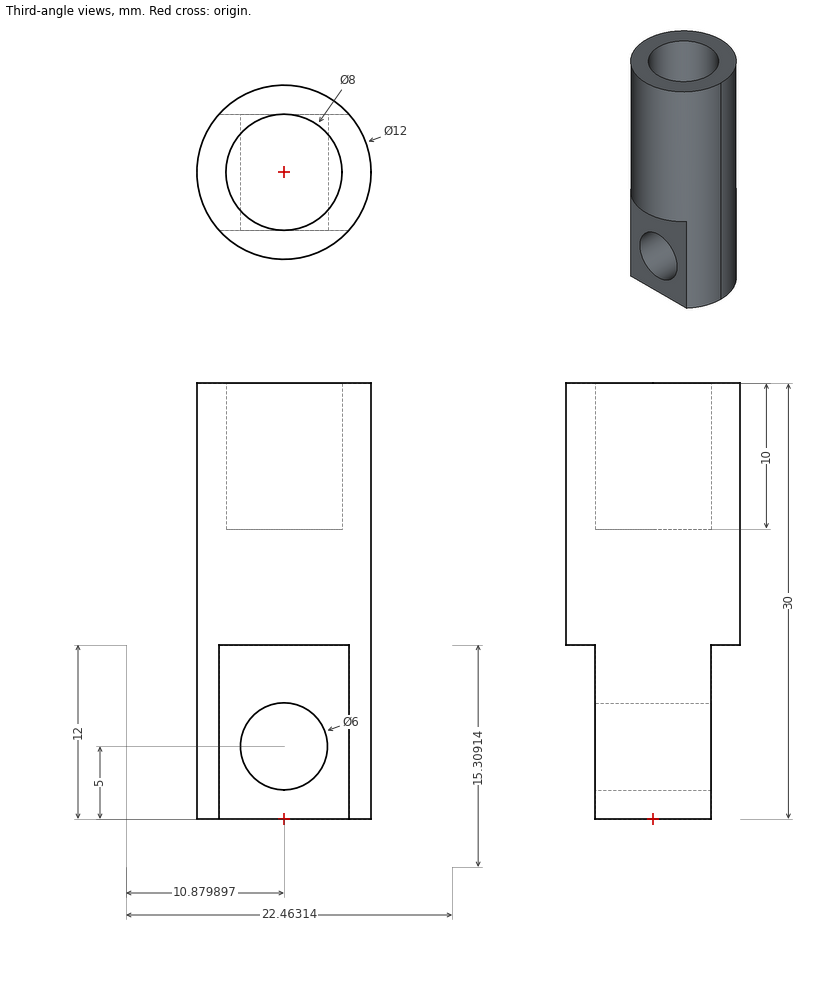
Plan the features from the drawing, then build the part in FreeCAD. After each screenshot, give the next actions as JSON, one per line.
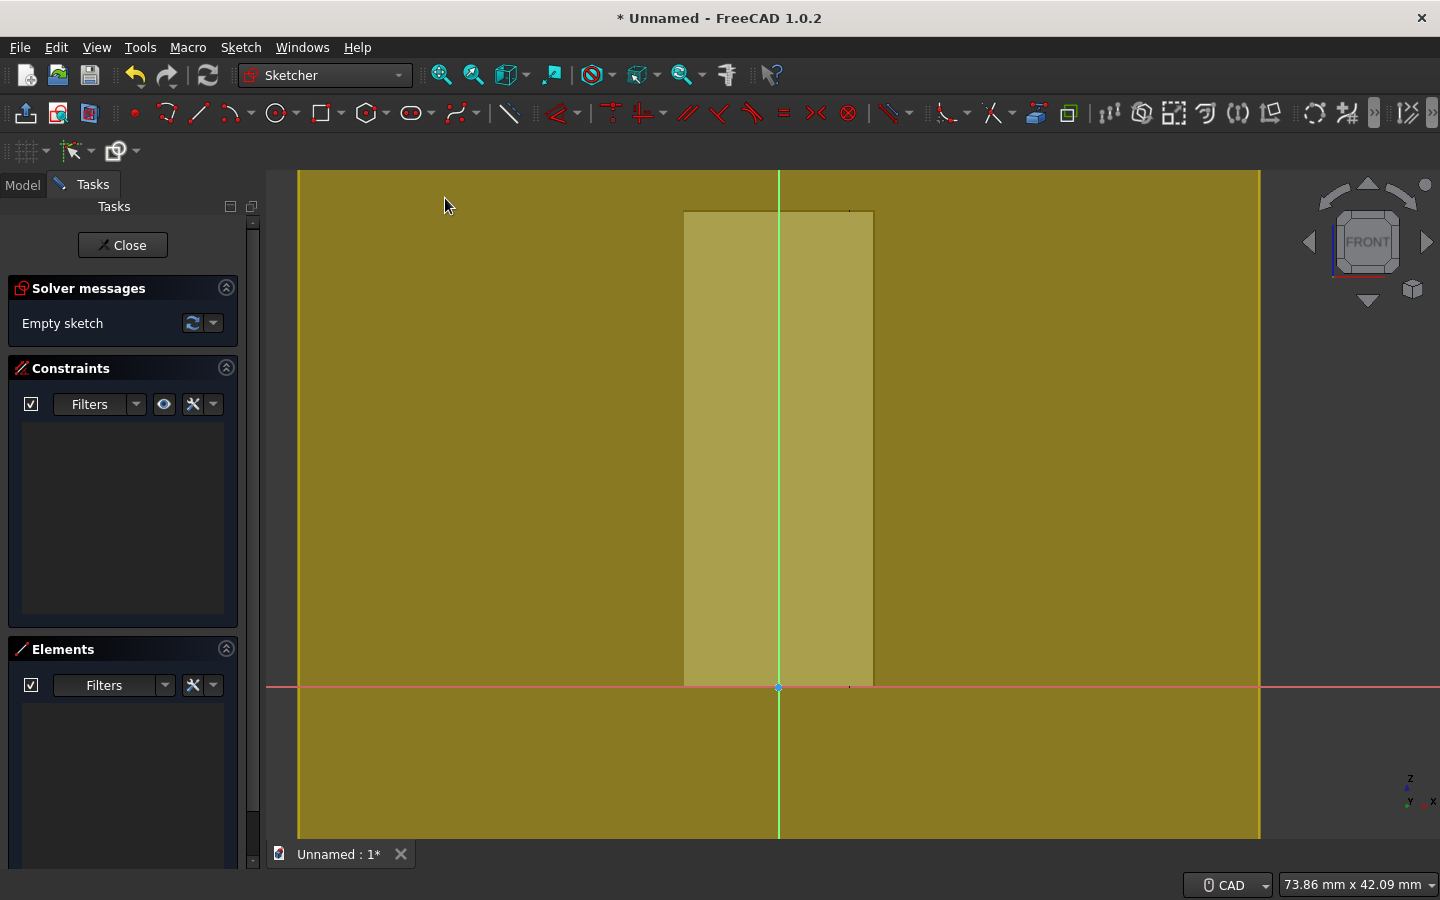
{"action": "scroll", "coordinate": [785, 757], "scroll_direction": "up", "scroll_amount": 3}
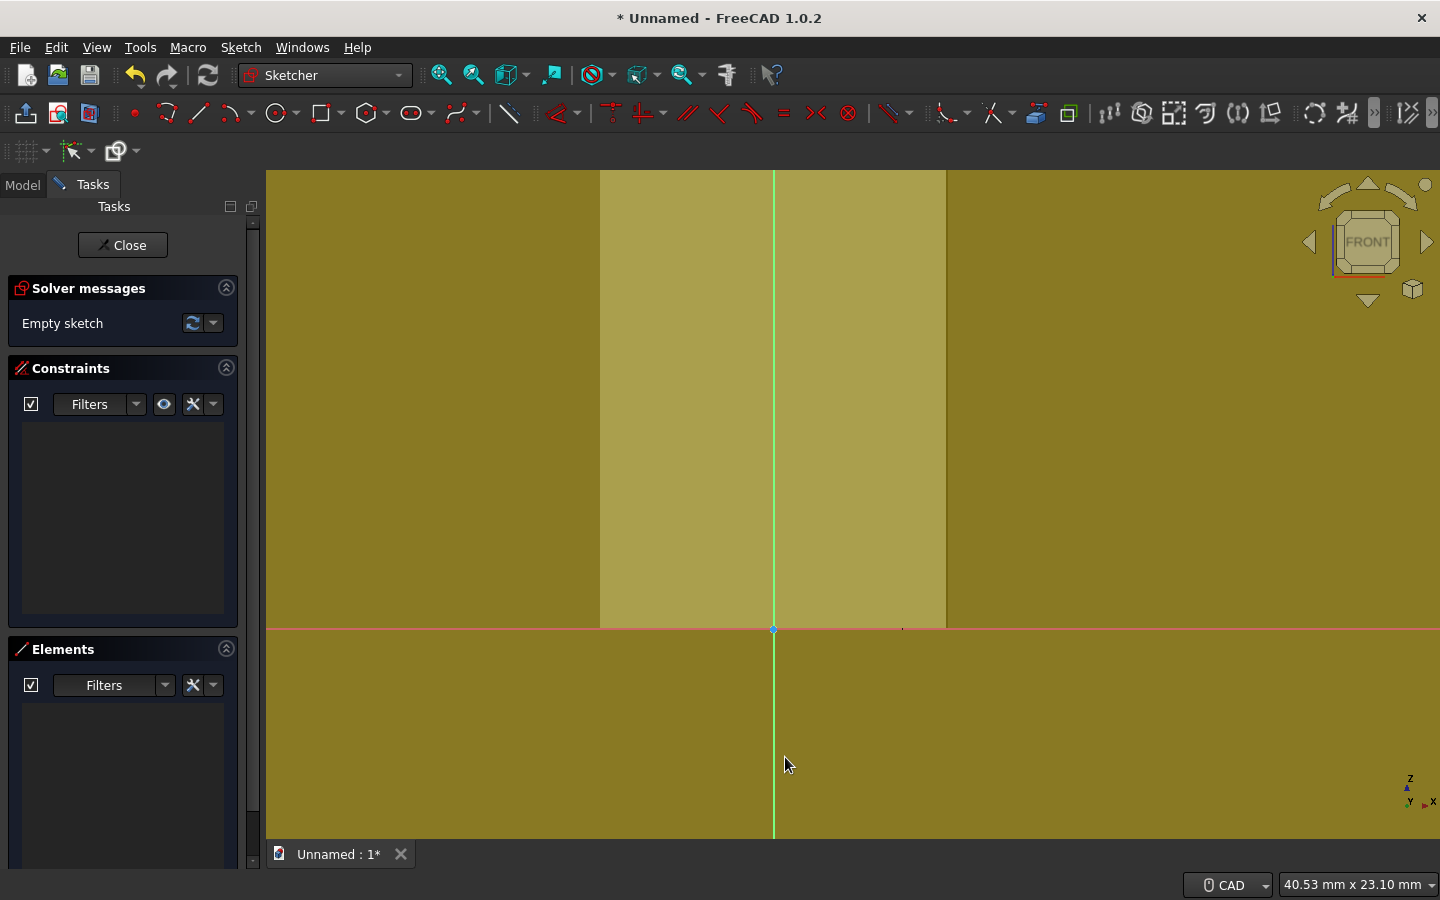
{"action": "left_click", "coordinate": [322, 114]}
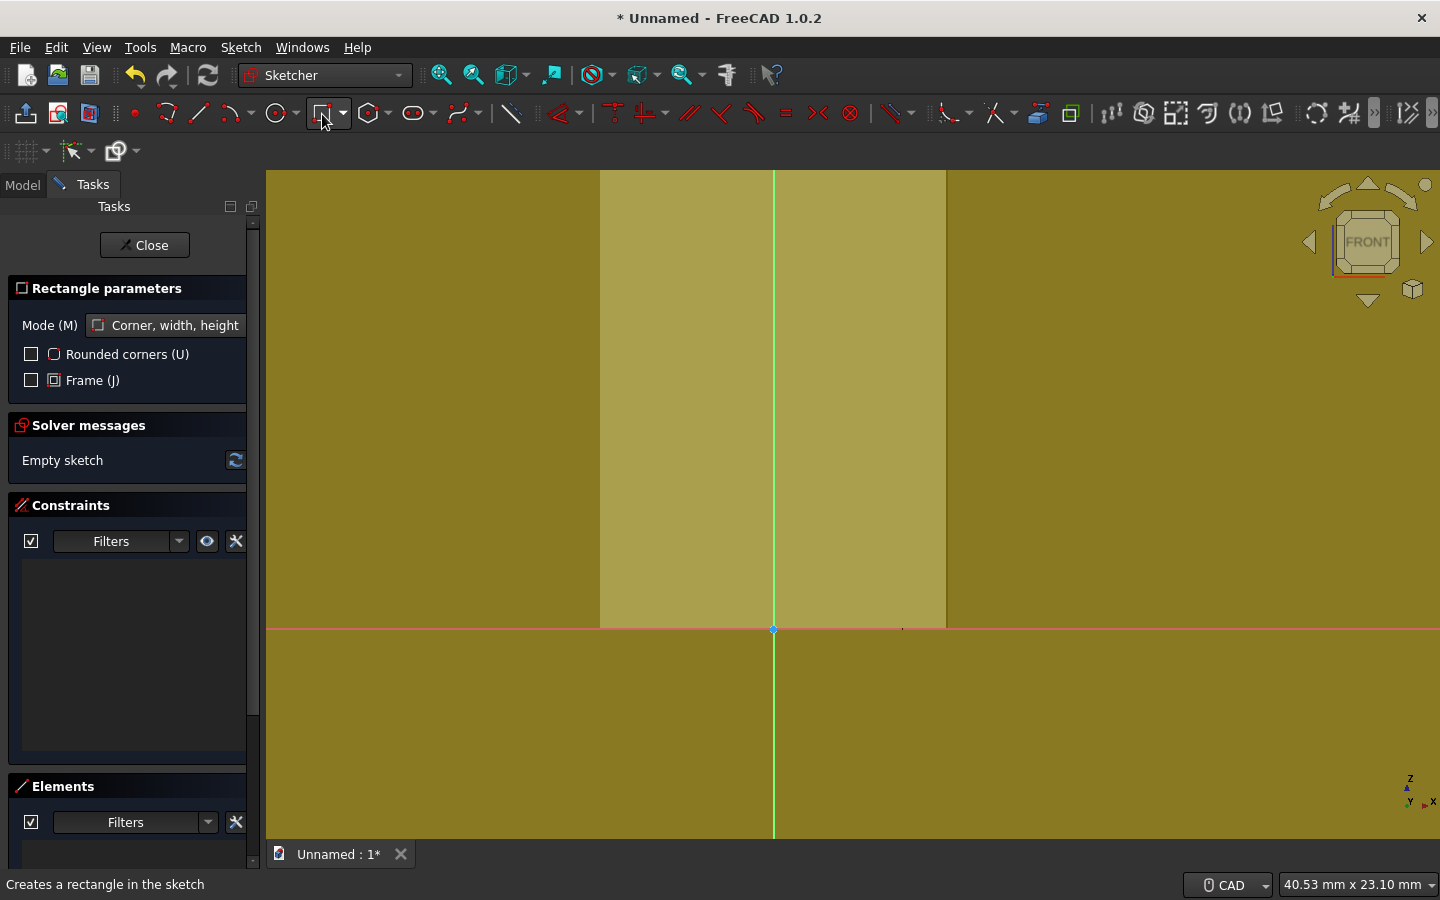
{"action": "left_click", "coordinate": [458, 282]}
{"action": "mouse_move", "coordinate": [1109, 725]}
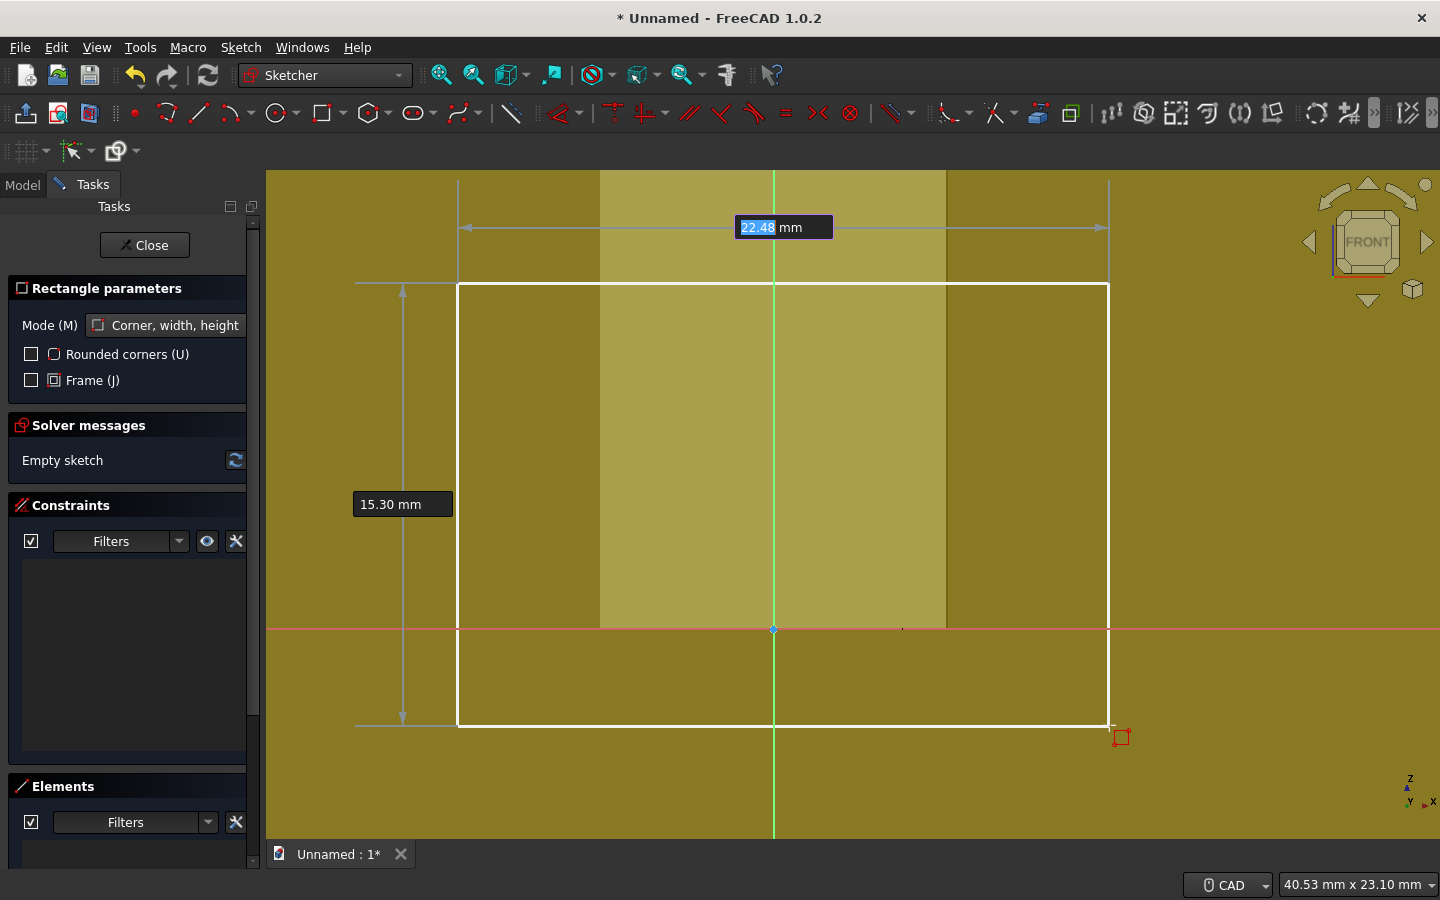
{"action": "type", "text": "22.46314"}
{"action": "key", "text": "Tab"}
{"action": "type", "text": "15.30914"}
{"action": "key", "text": "Return"}
{"action": "key", "text": "Escape"}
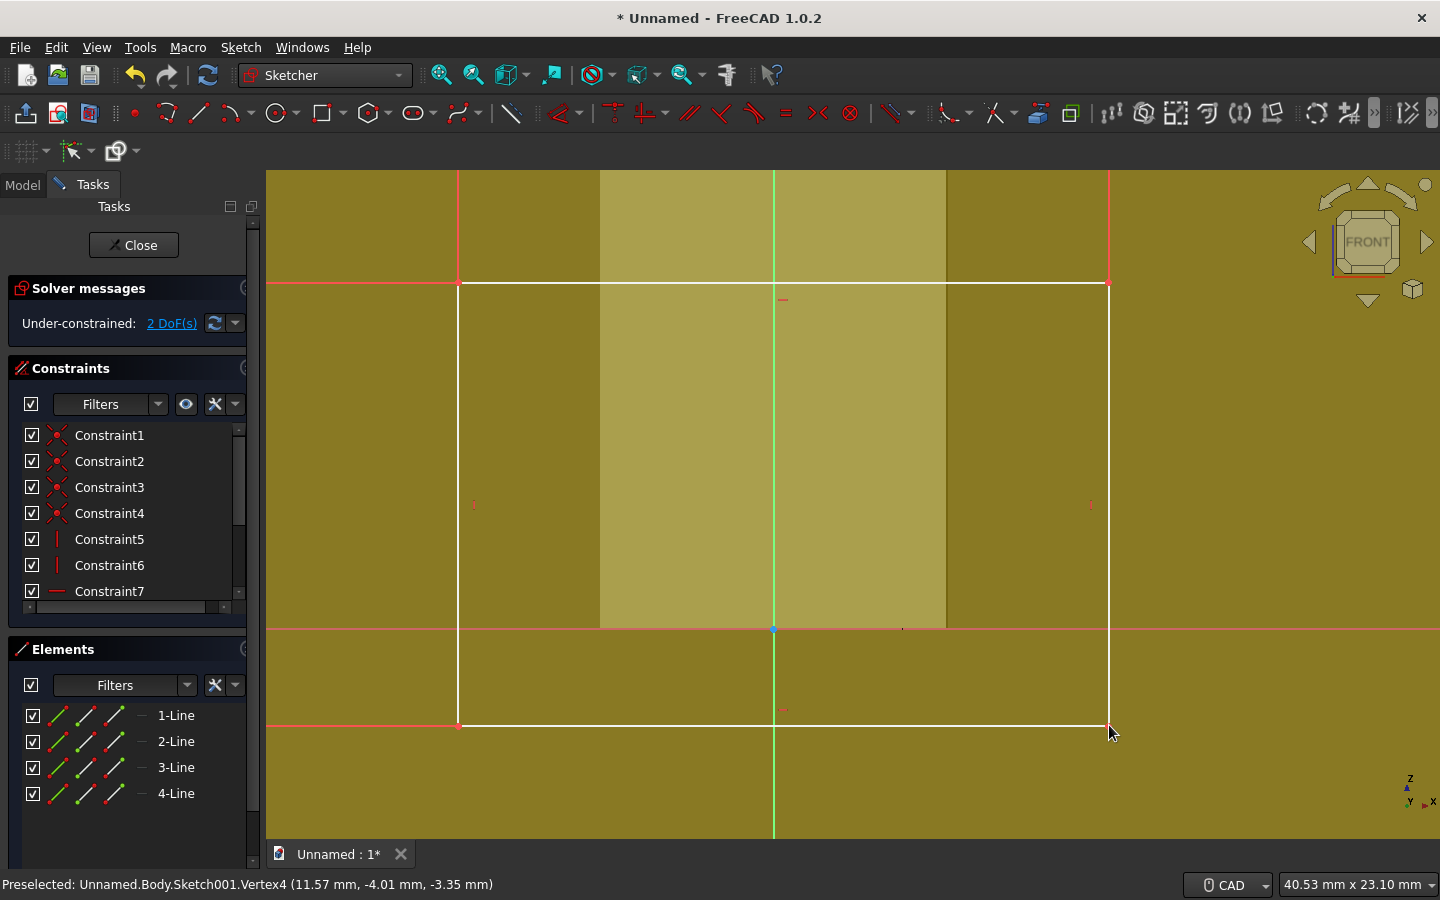
{"action": "left_click", "coordinate": [558, 114]}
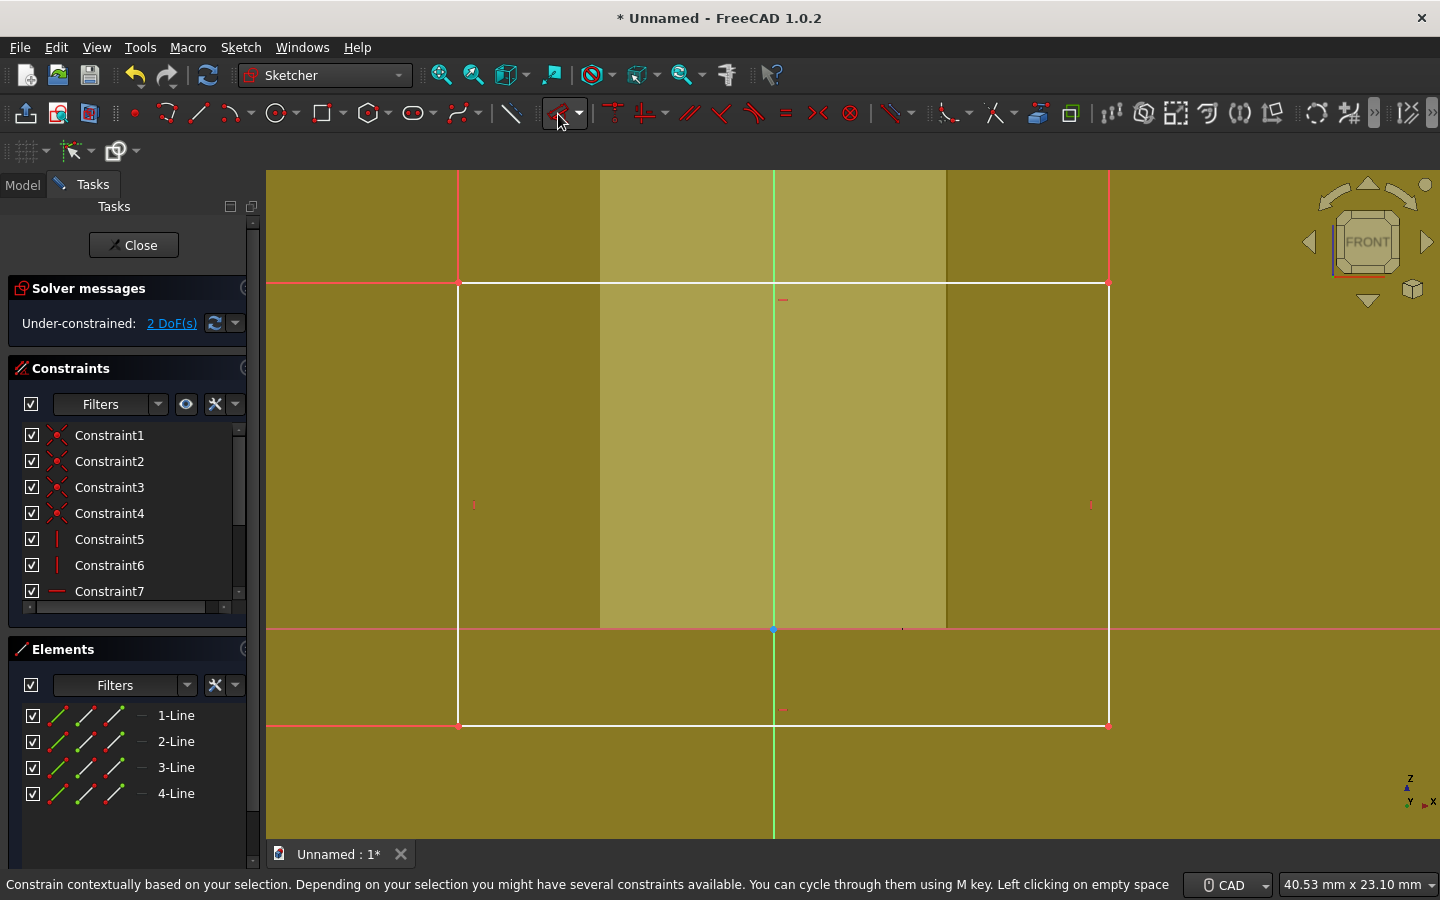
{"action": "left_click", "coordinate": [458, 283]}
{"action": "left_click", "coordinate": [424, 456]}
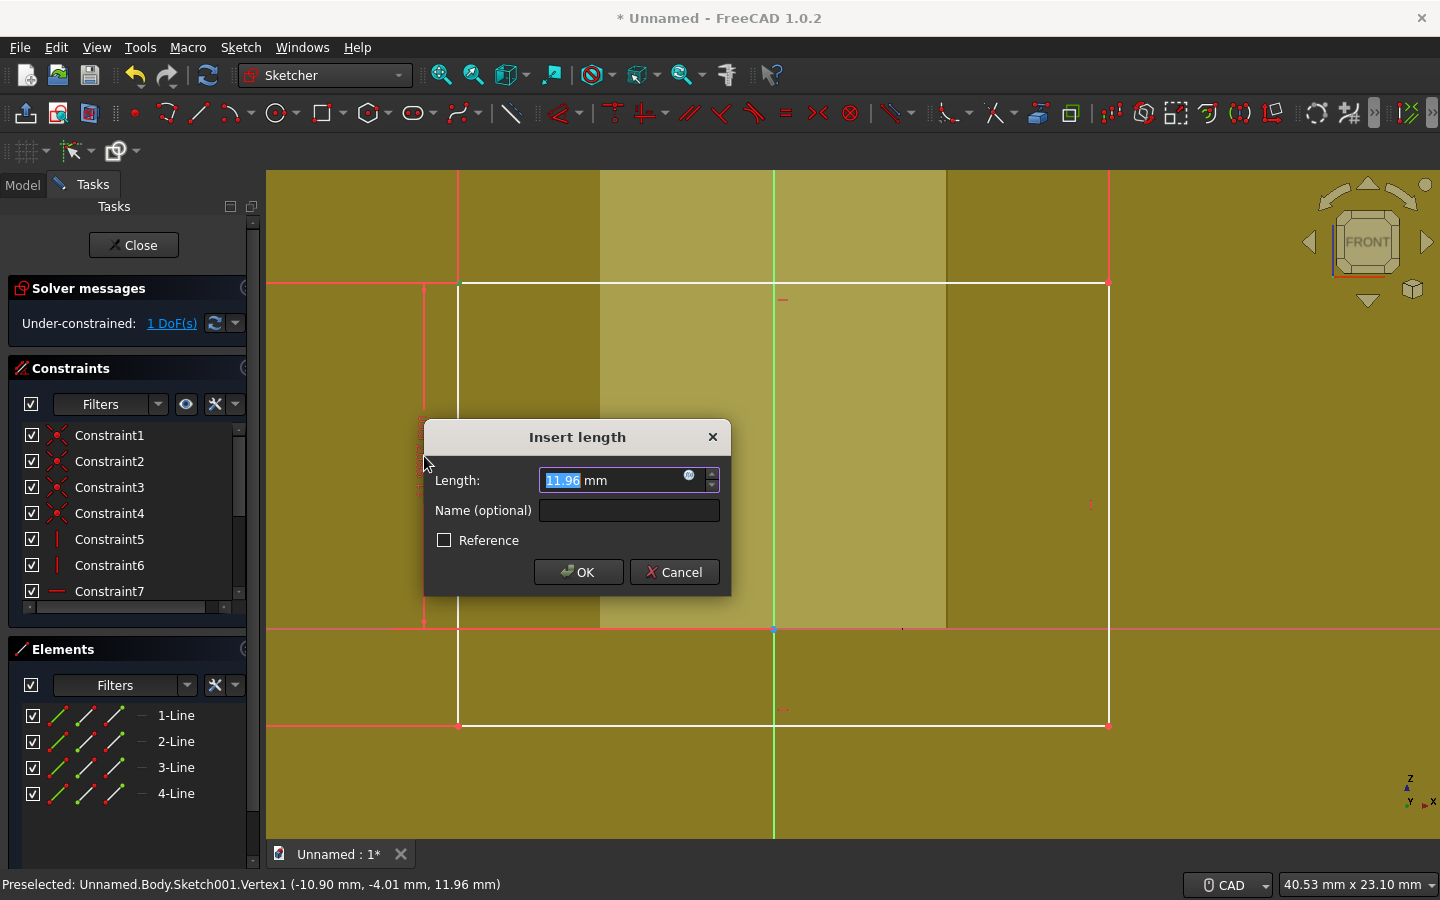
{"action": "type", "text": "12"}
{"action": "key", "text": "Return"}